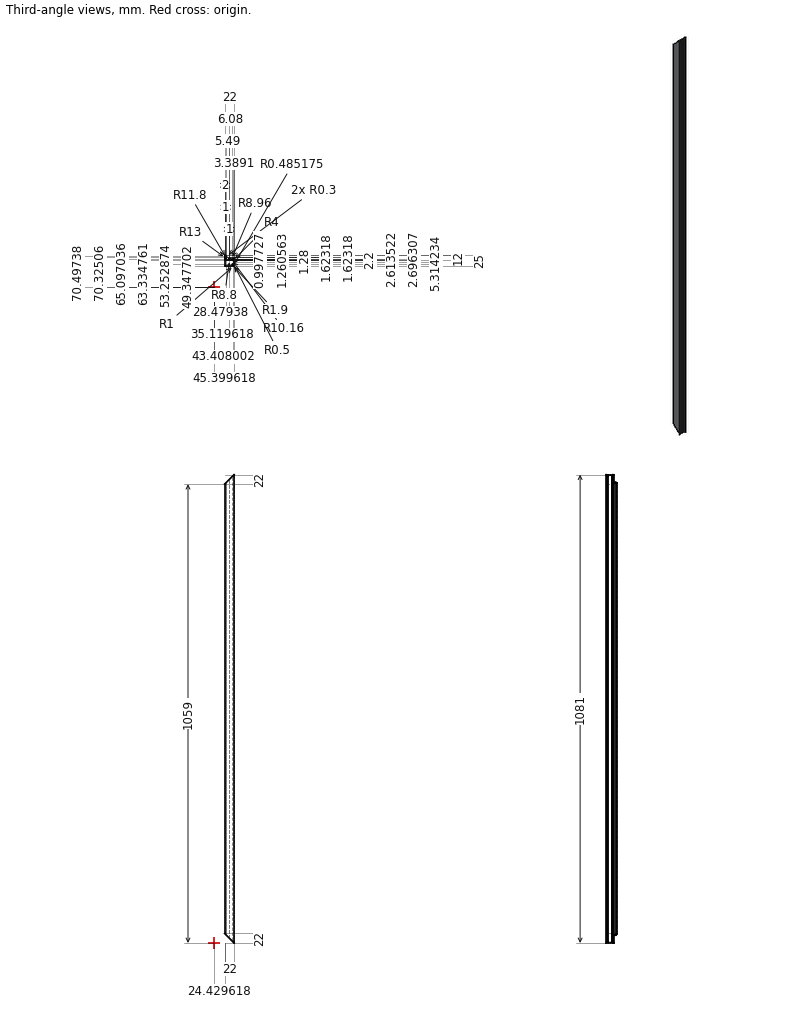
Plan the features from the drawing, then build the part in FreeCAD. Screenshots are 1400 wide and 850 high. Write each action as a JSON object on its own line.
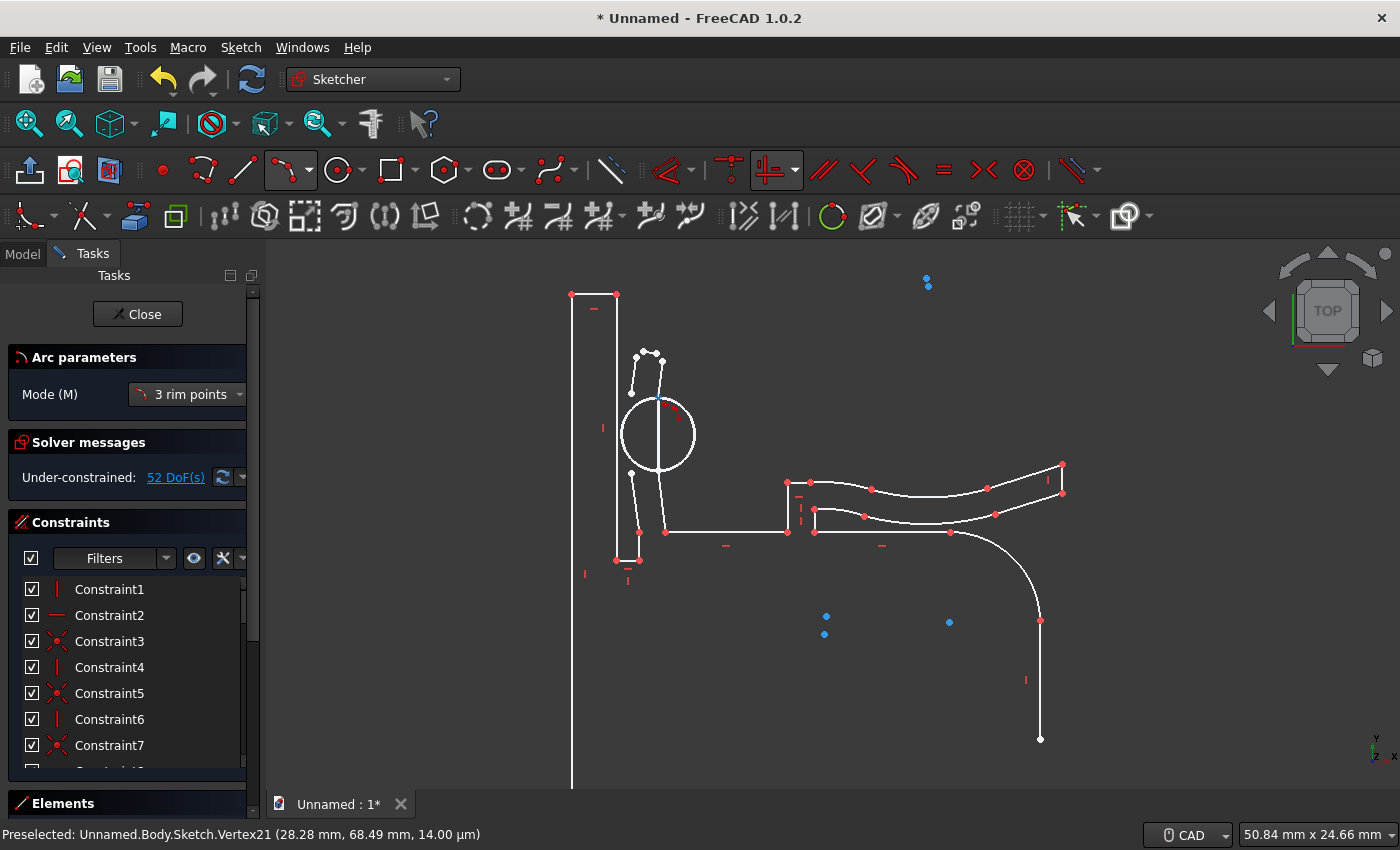
{"action": "scroll", "coordinate": [655, 433], "scroll_direction": "up", "scroll_amount": 10}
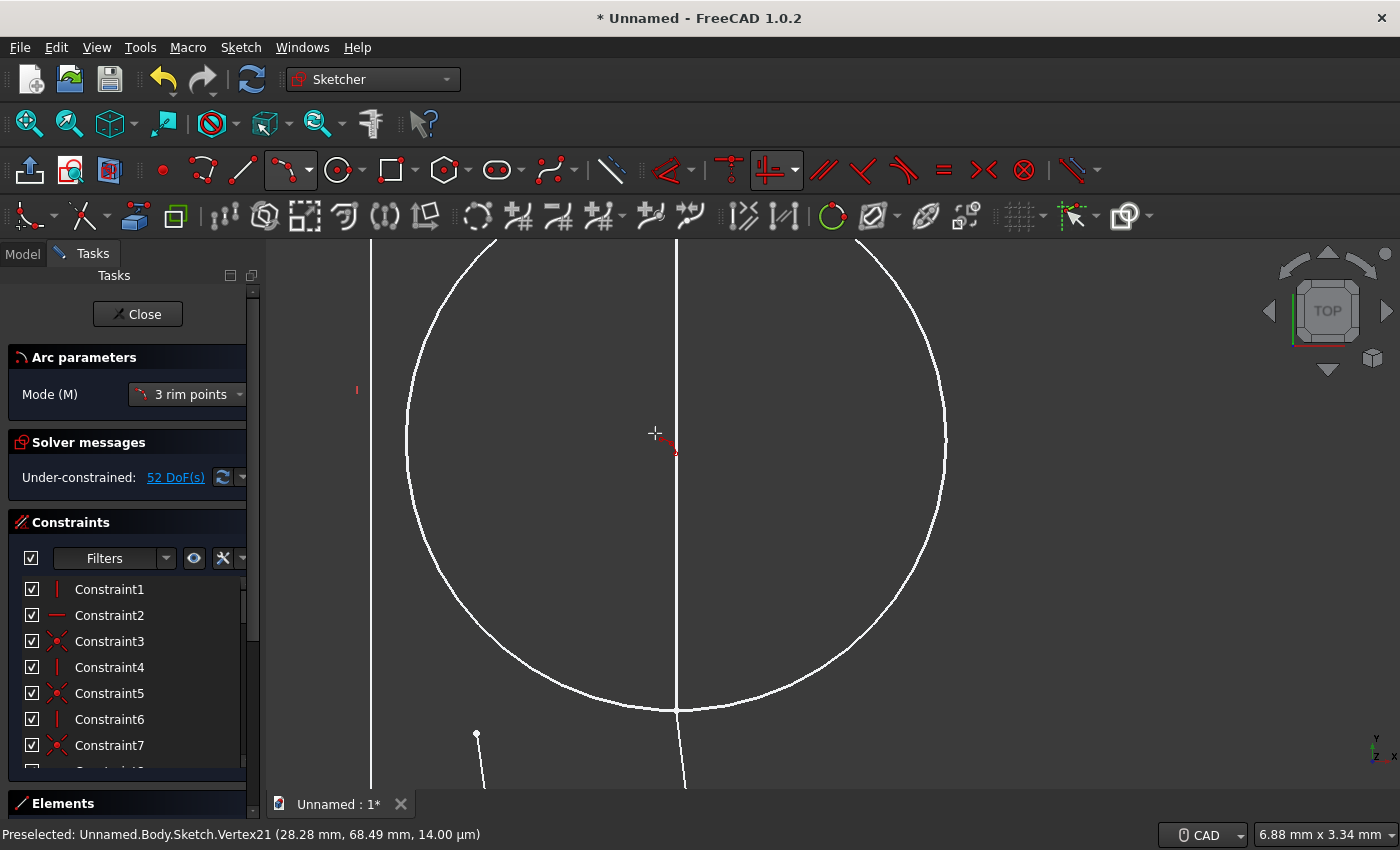
{"action": "left_click", "coordinate": [653, 433]}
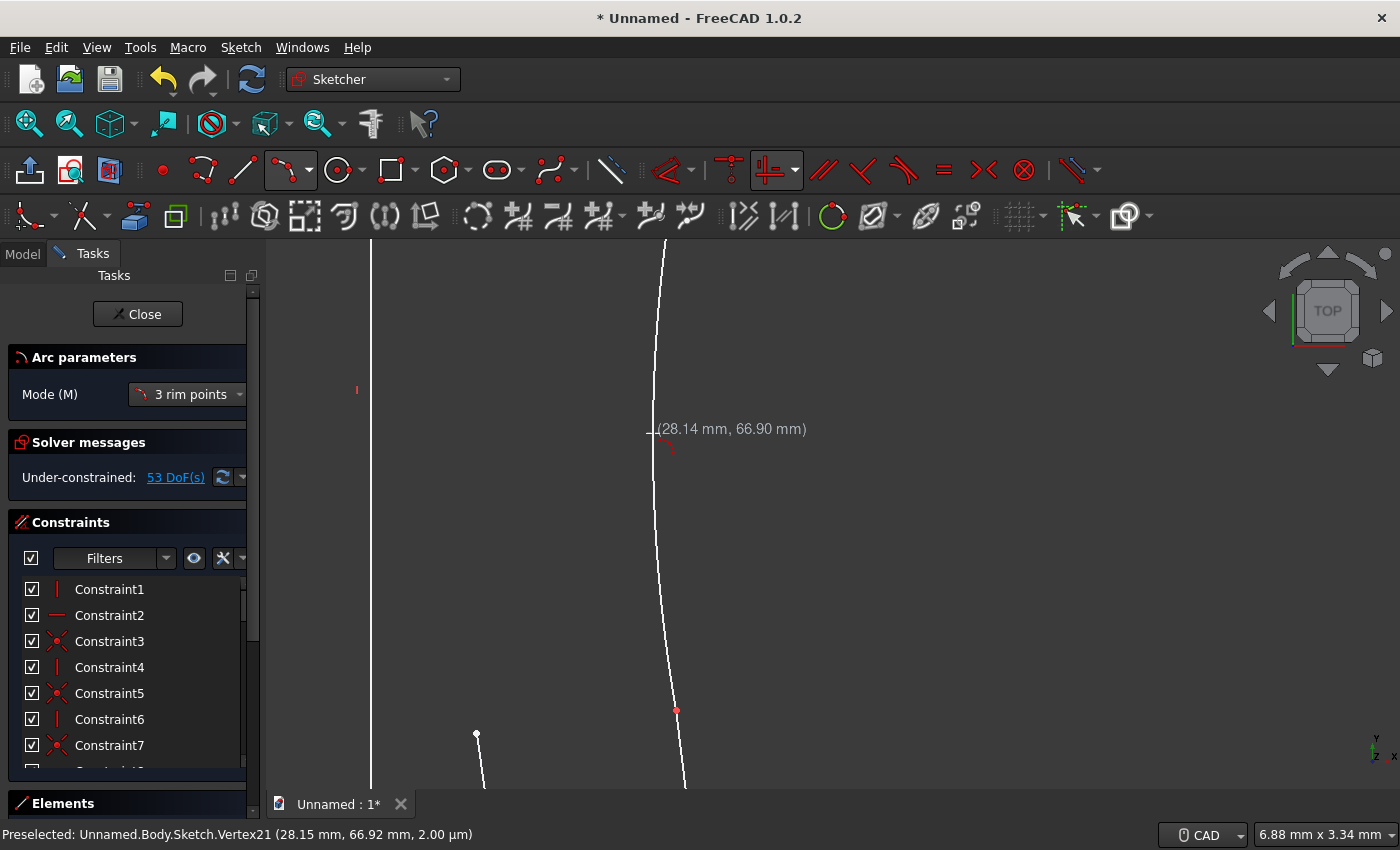
{"action": "scroll", "coordinate": [656, 420], "scroll_direction": "down", "scroll_amount": 12}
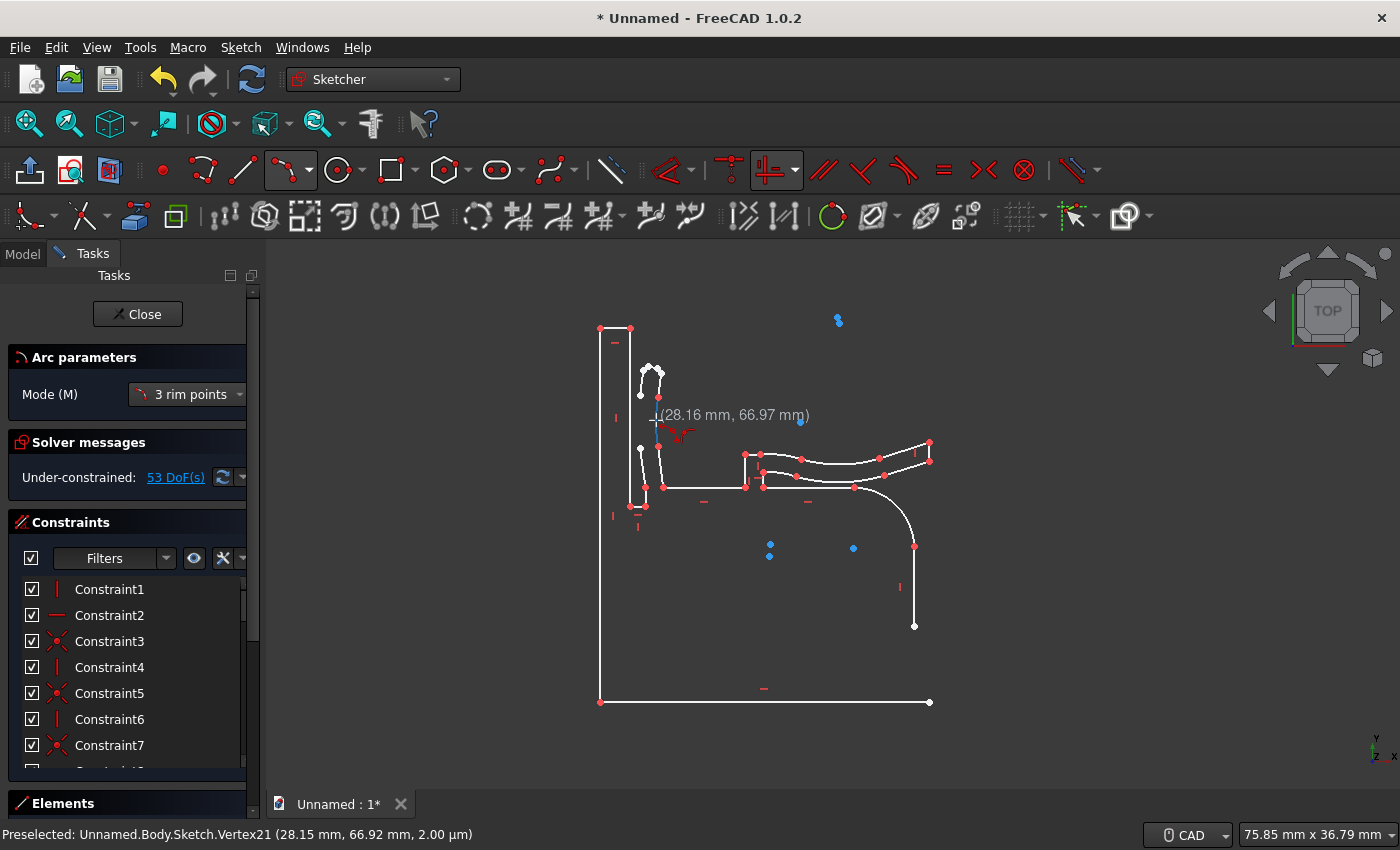
{"action": "scroll", "coordinate": [661, 373], "scroll_direction": "up", "scroll_amount": 5}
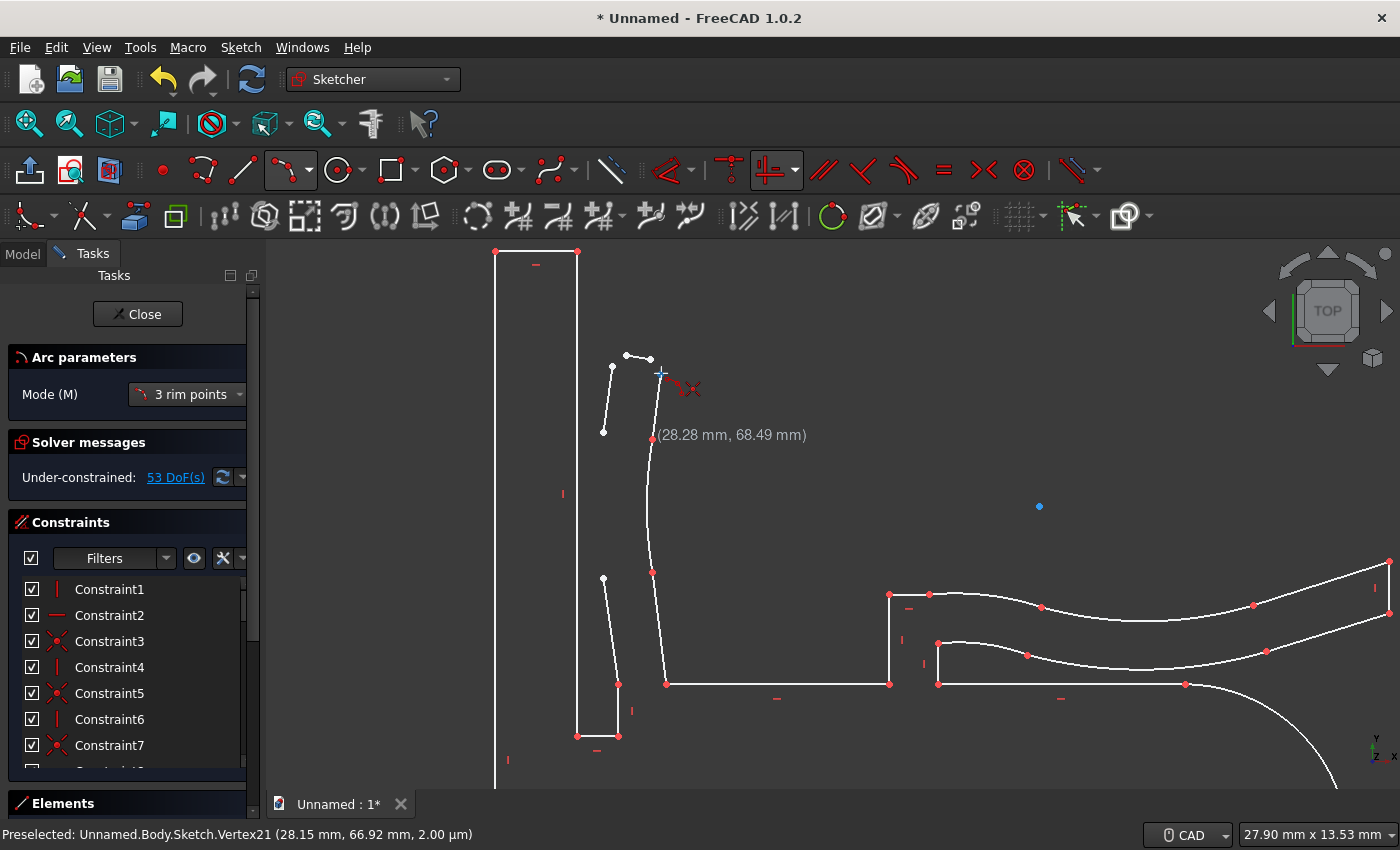
{"action": "left_click", "coordinate": [661, 374]}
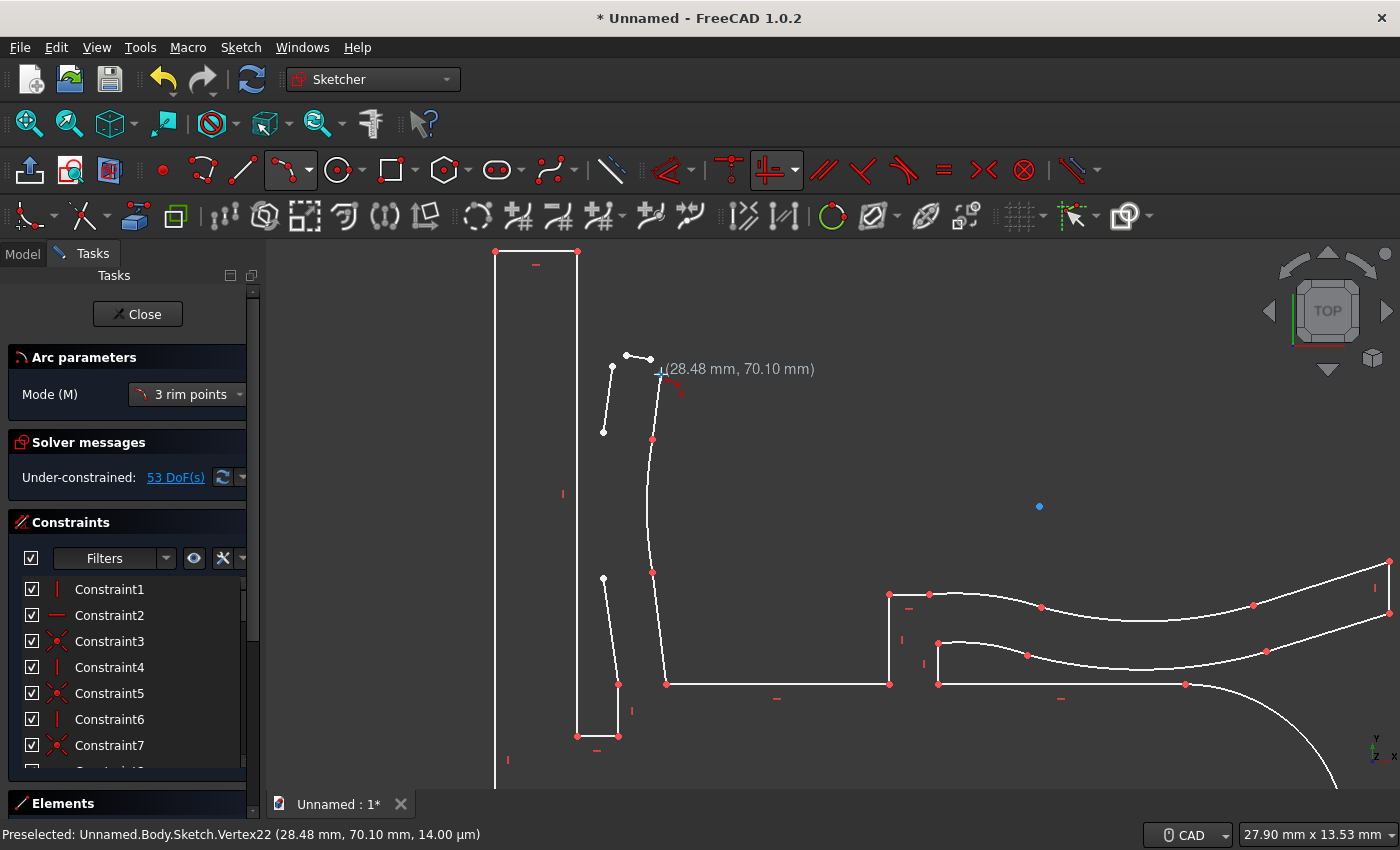
{"action": "scroll", "coordinate": [650, 358], "scroll_direction": "up", "scroll_amount": 2}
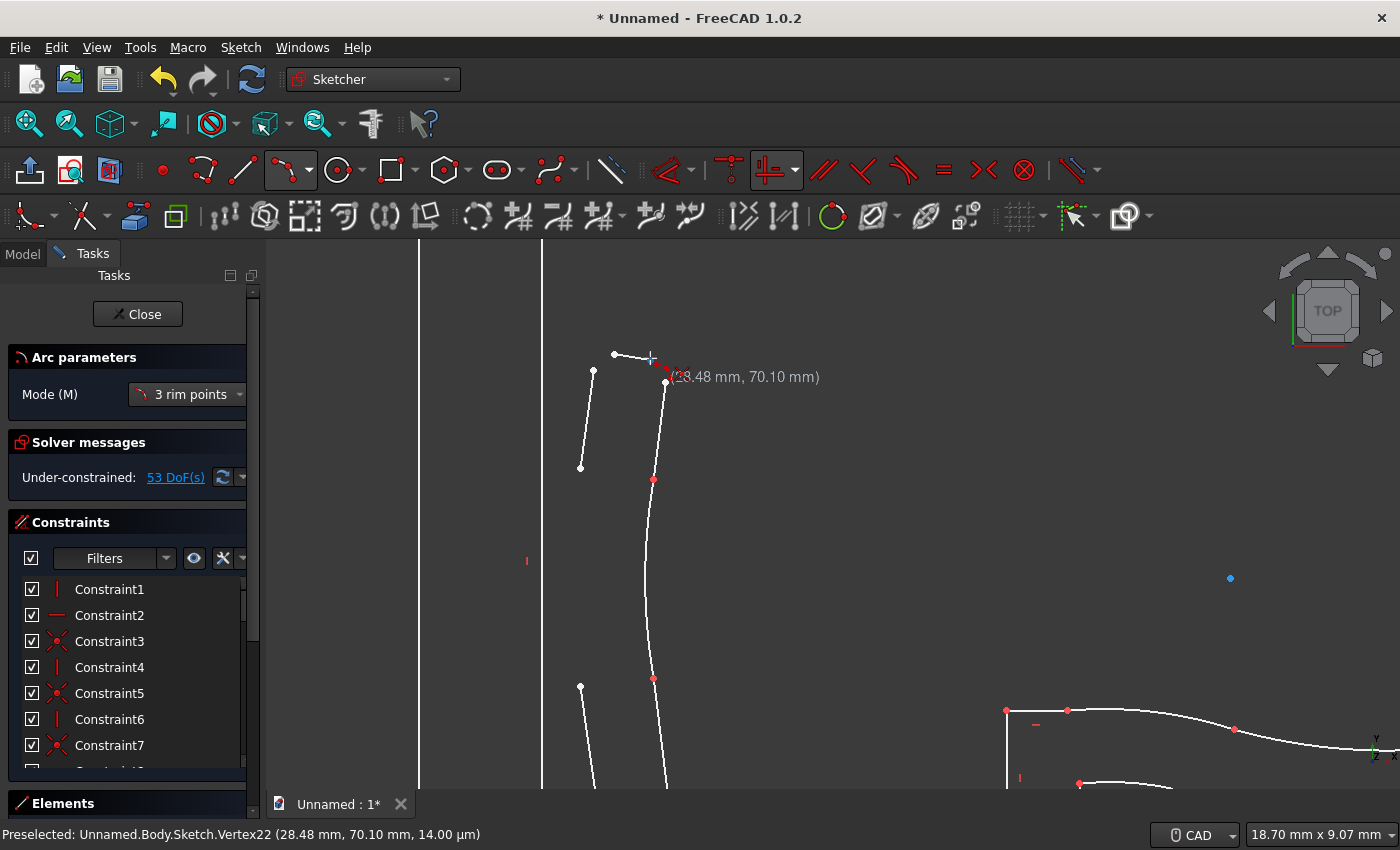
{"action": "left_click", "coordinate": [651, 360]}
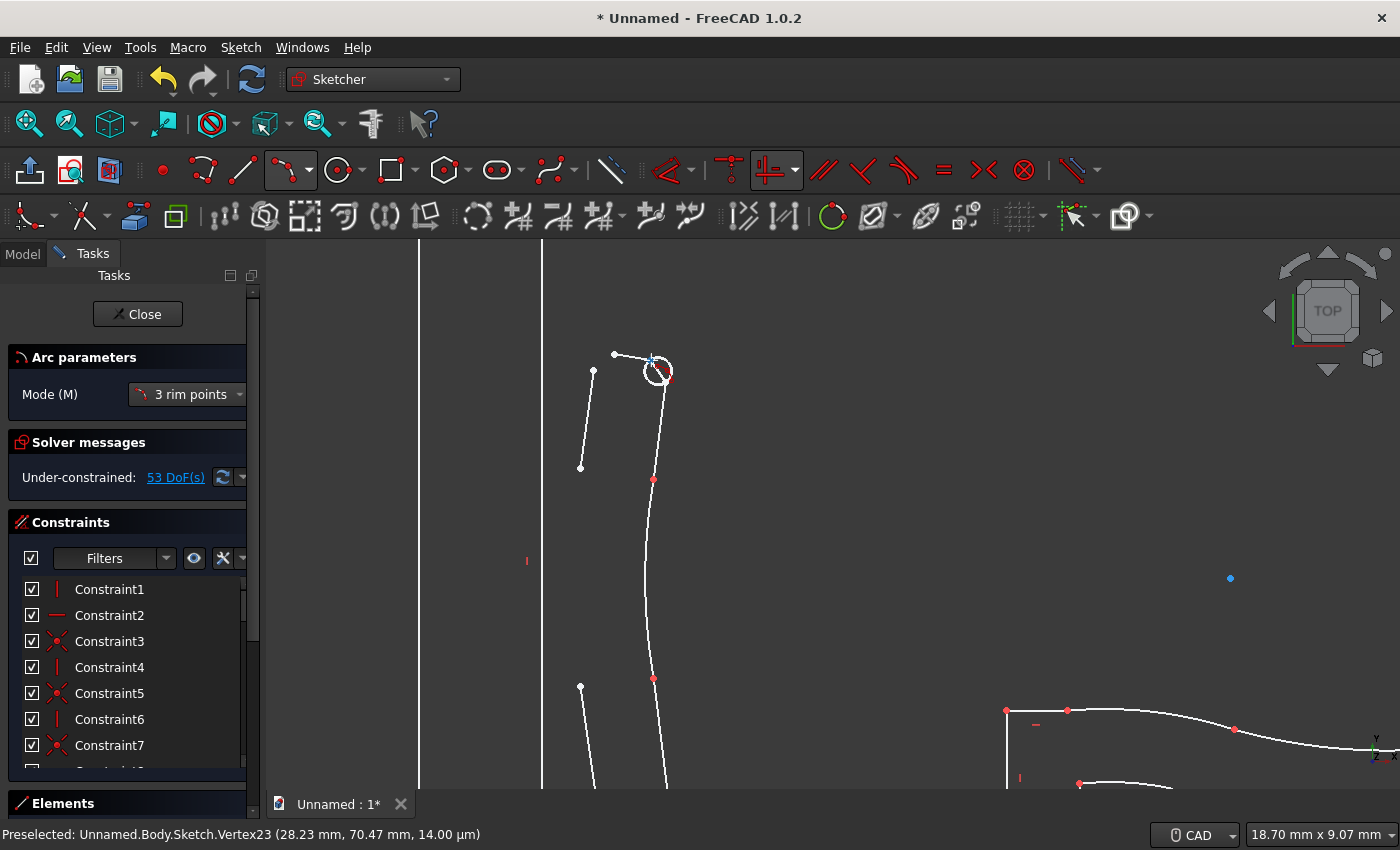
{"action": "scroll", "coordinate": [662, 365], "scroll_direction": "up", "scroll_amount": 6}